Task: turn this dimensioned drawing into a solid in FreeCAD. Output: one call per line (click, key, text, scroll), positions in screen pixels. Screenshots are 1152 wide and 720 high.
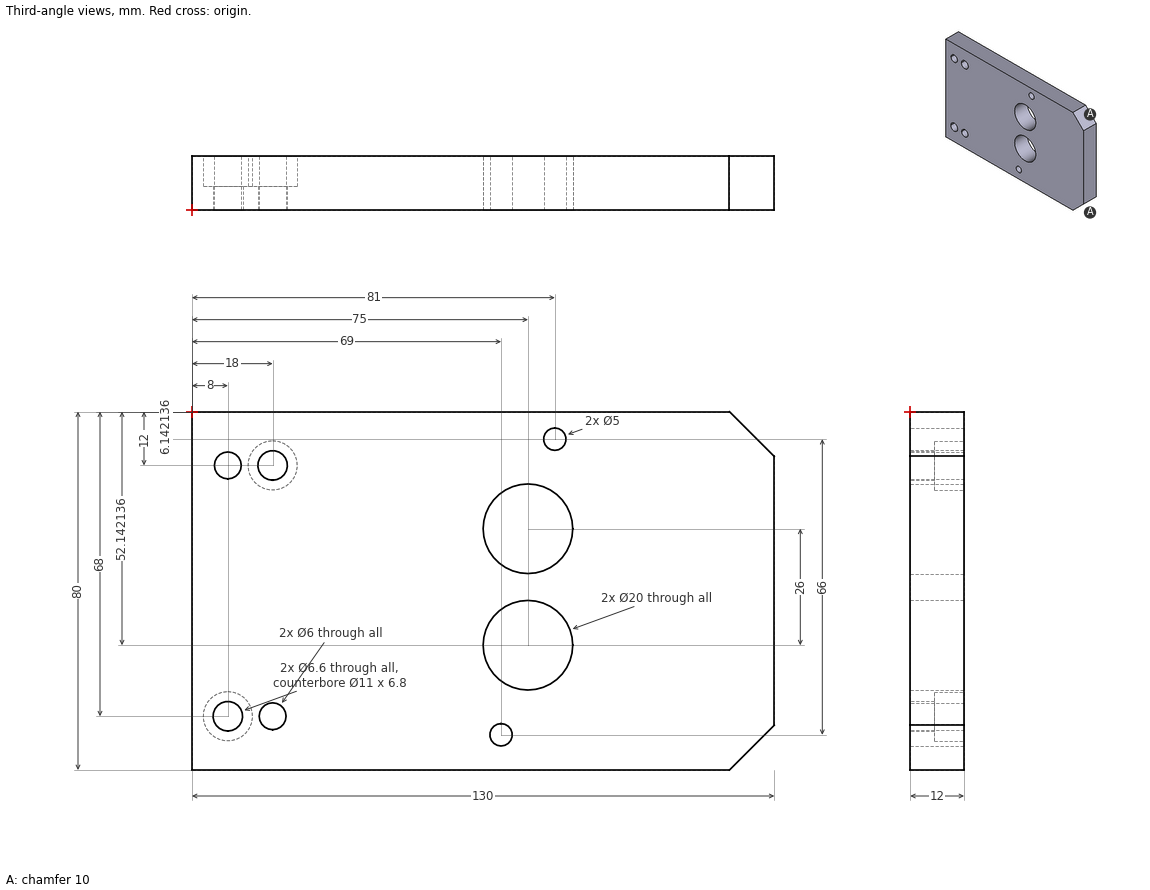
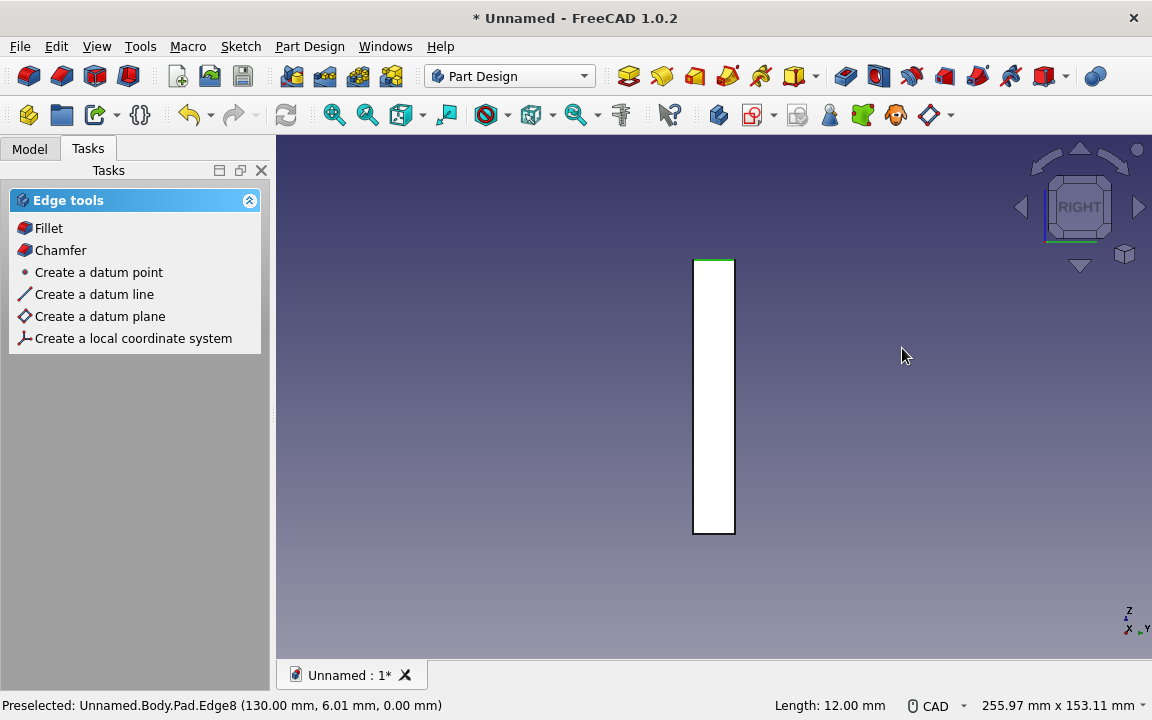
click(714, 533, ctrl)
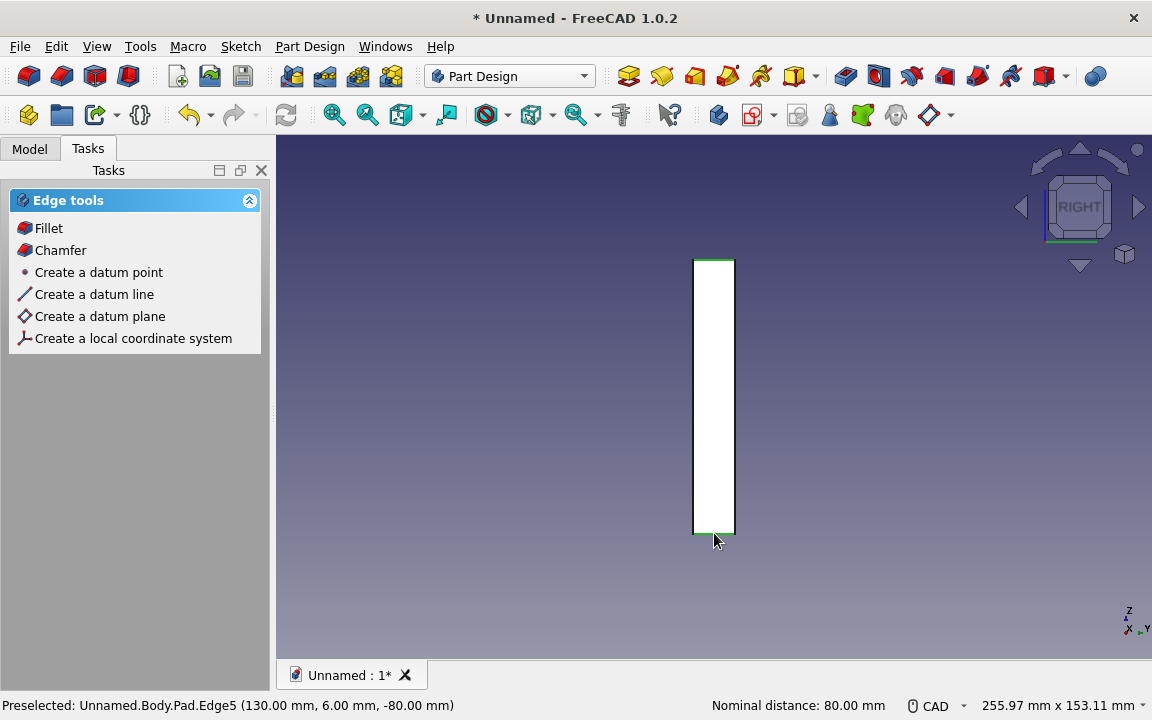
click(62, 76)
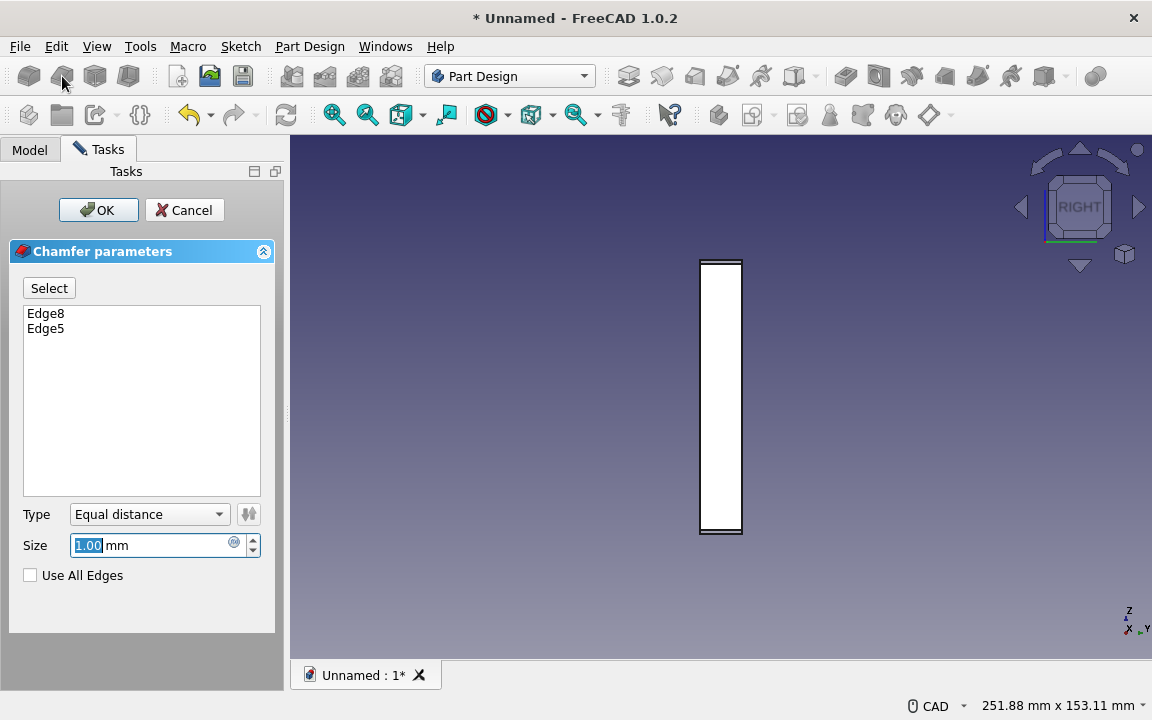
text(10)
key(Tab)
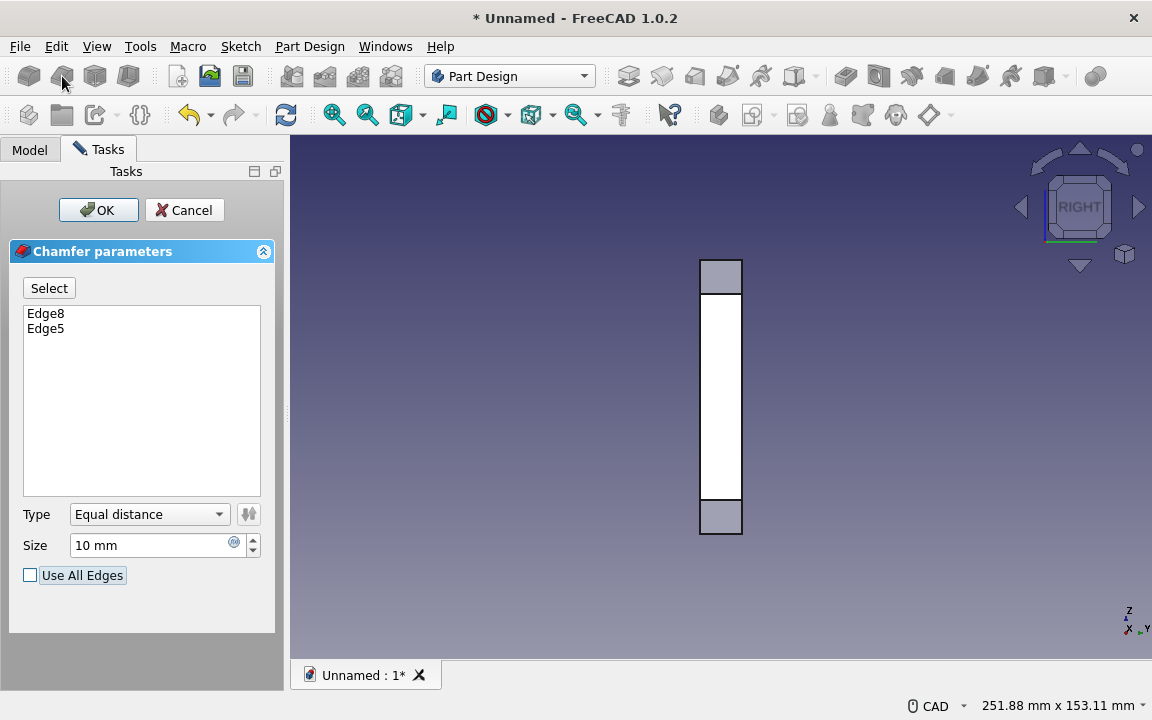
click(99, 210)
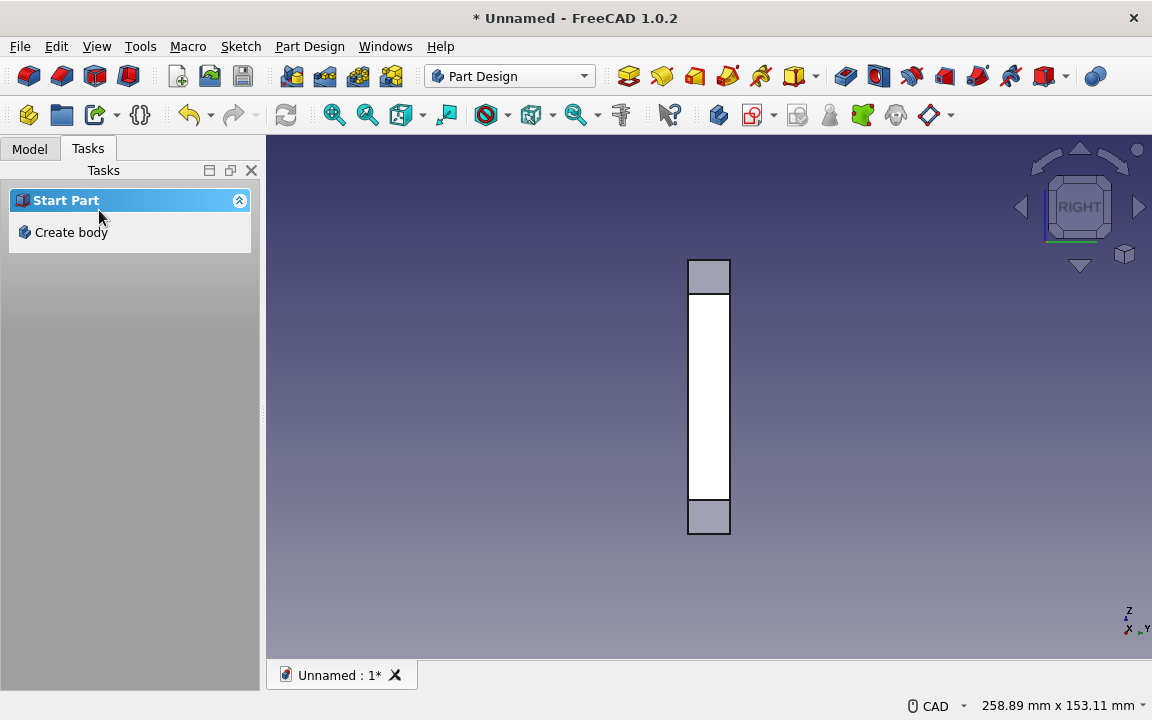
key(4)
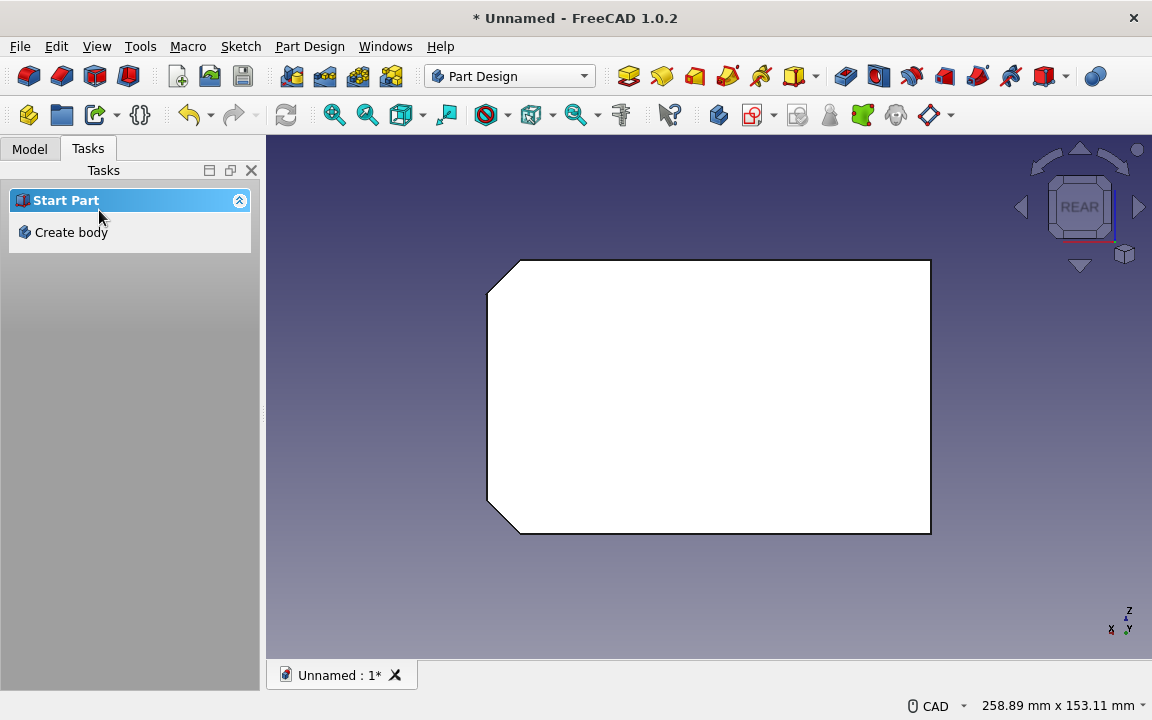
click(645, 396)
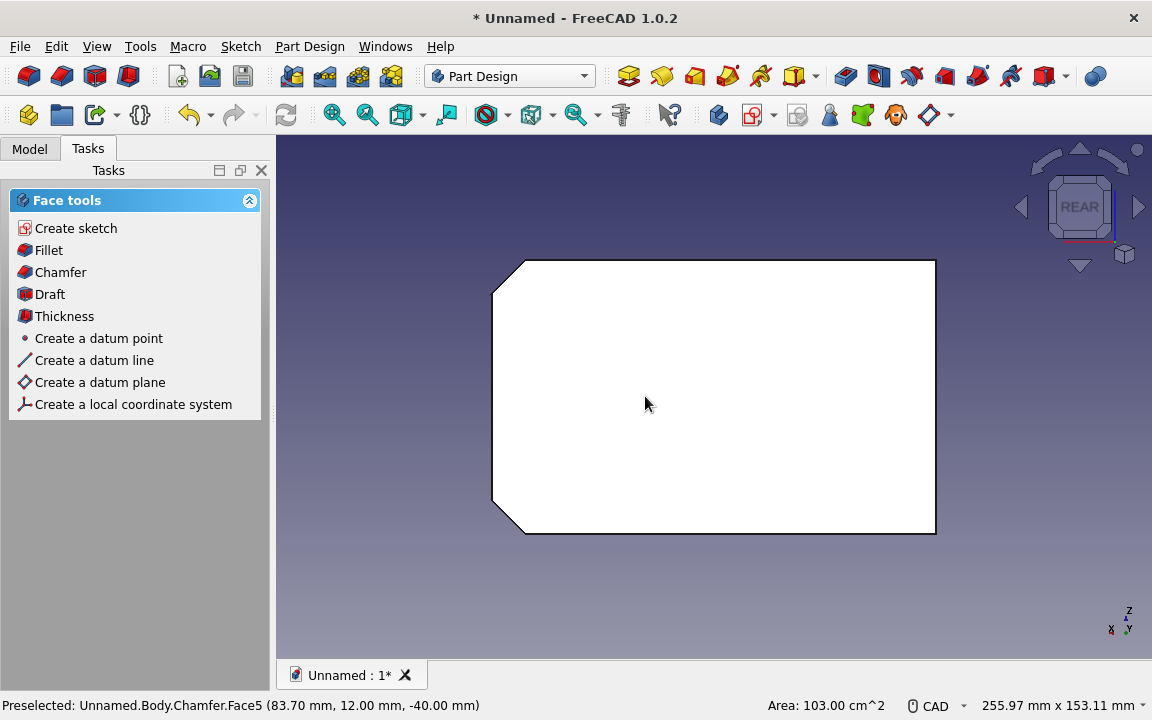
click(752, 116)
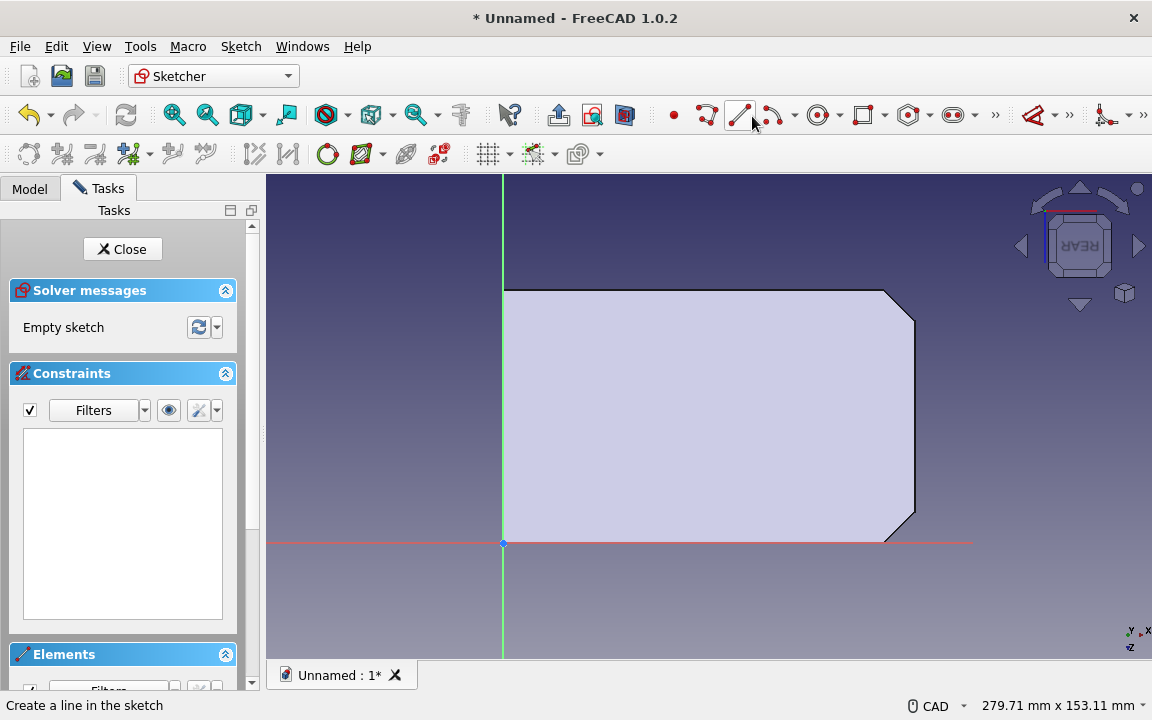
click(818, 116)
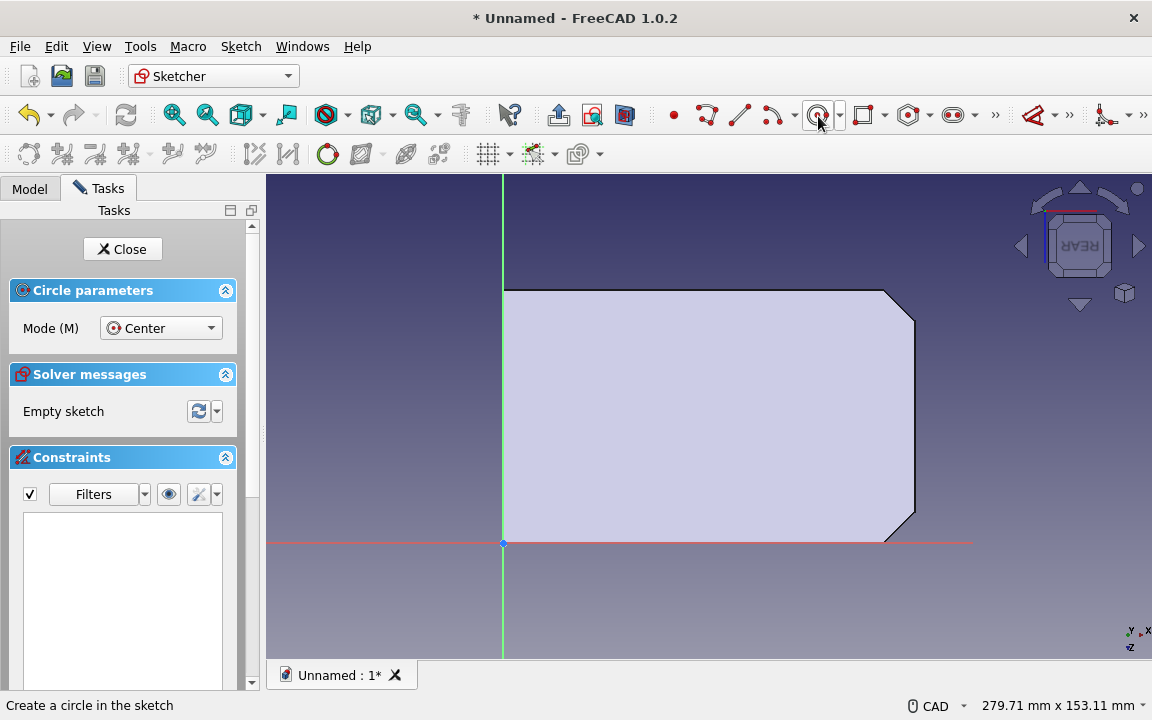
scroll(528, 328, up, 4)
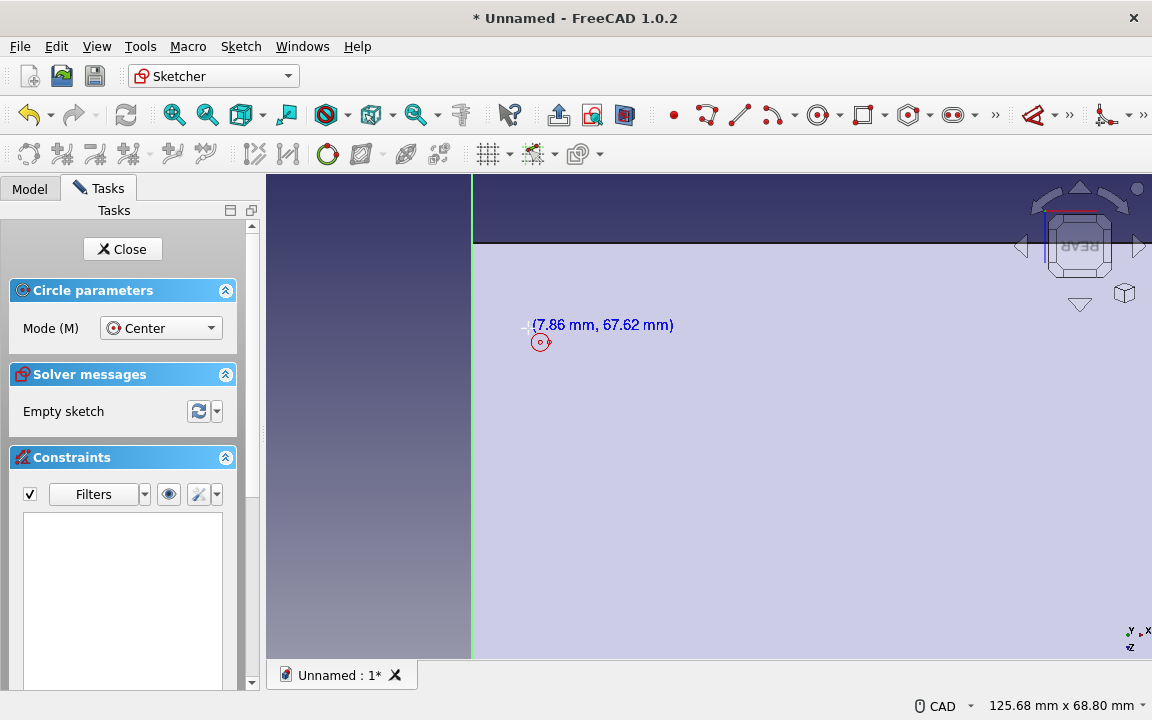
click(529, 327)
click(545, 311)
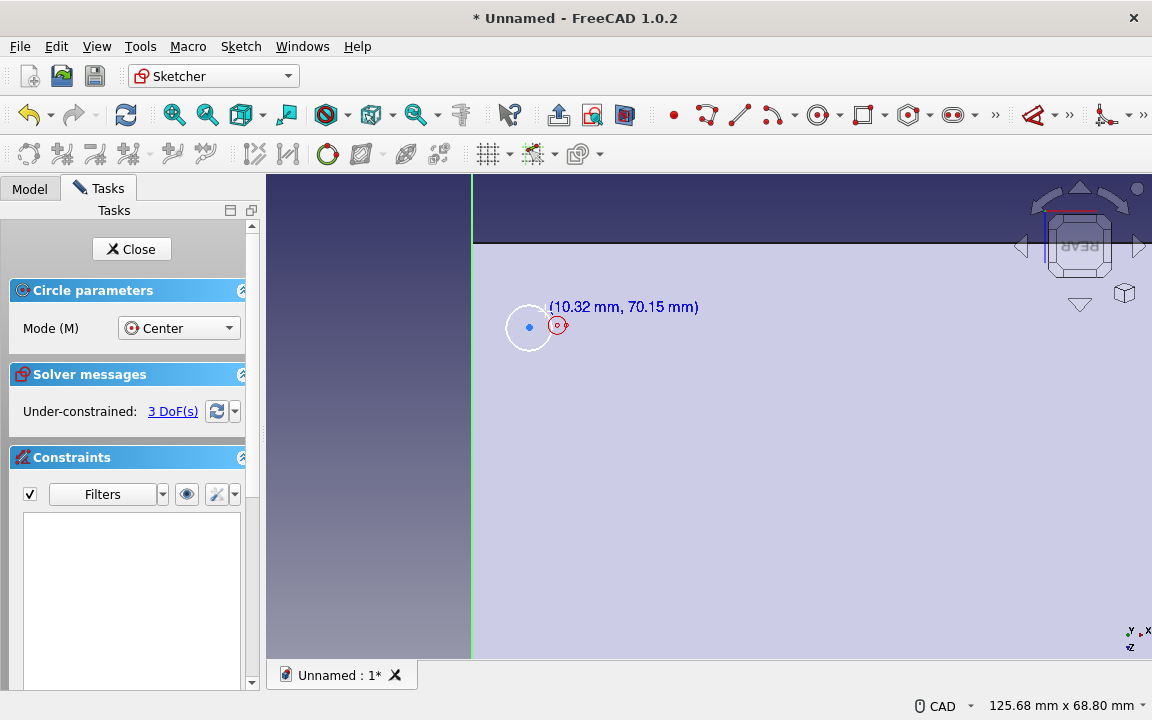
scroll(754, 248, down, 3)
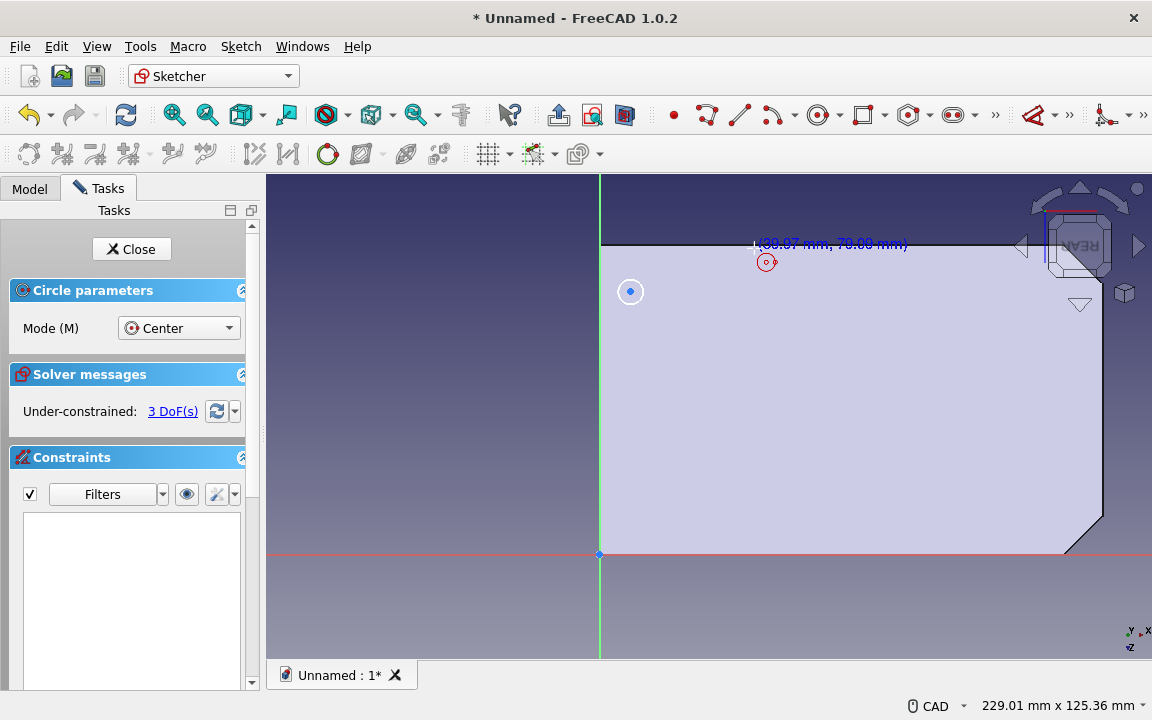
scroll(669, 508, up, 3)